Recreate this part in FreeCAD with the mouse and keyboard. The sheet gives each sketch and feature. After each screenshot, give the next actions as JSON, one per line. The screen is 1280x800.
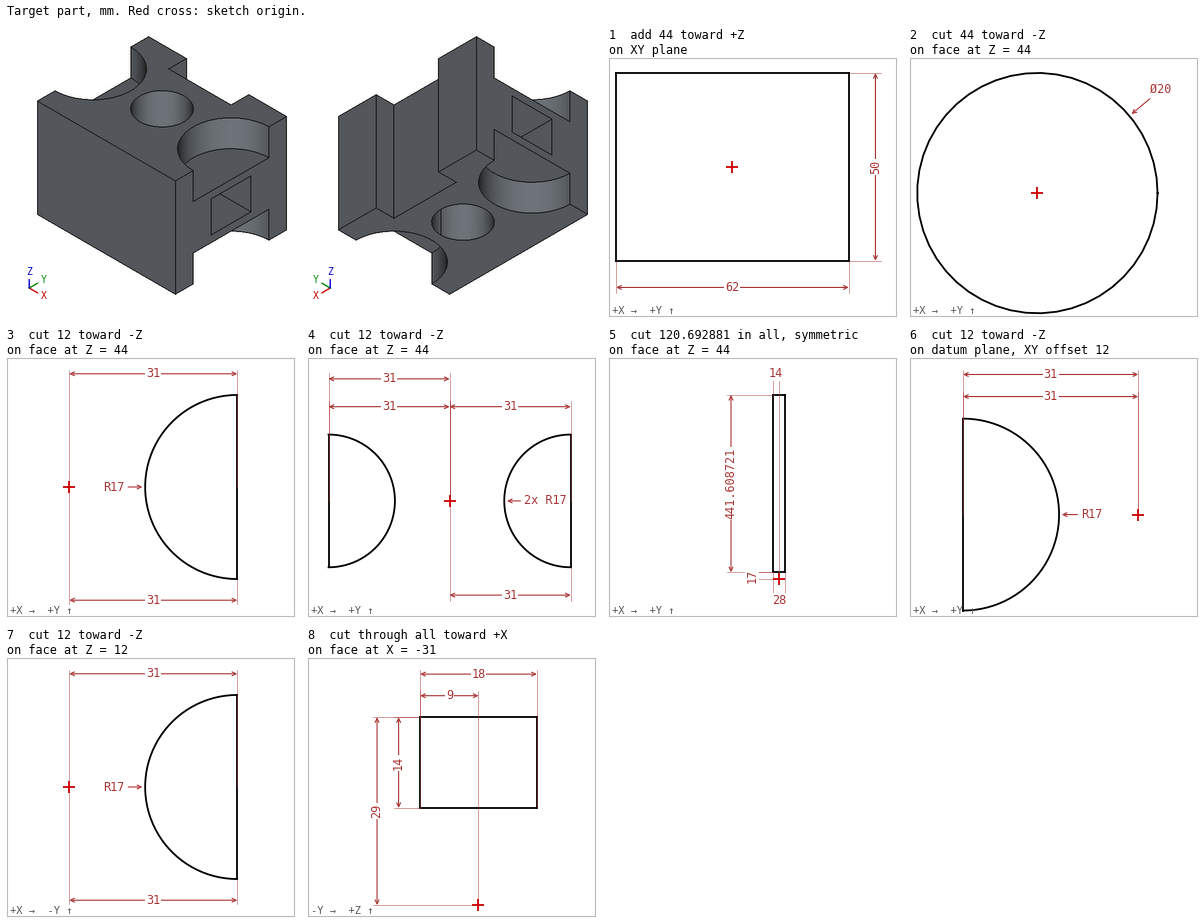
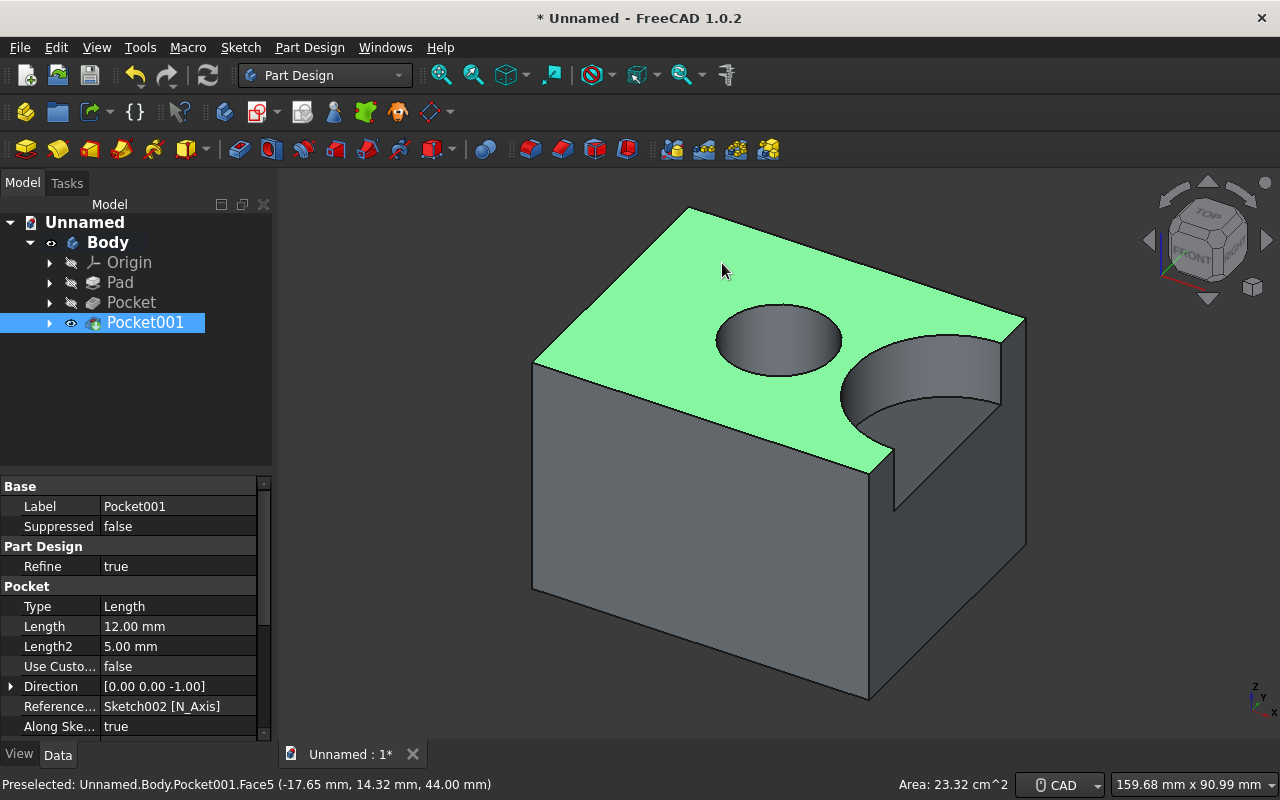
{"action": "left_click", "coordinate": [258, 112]}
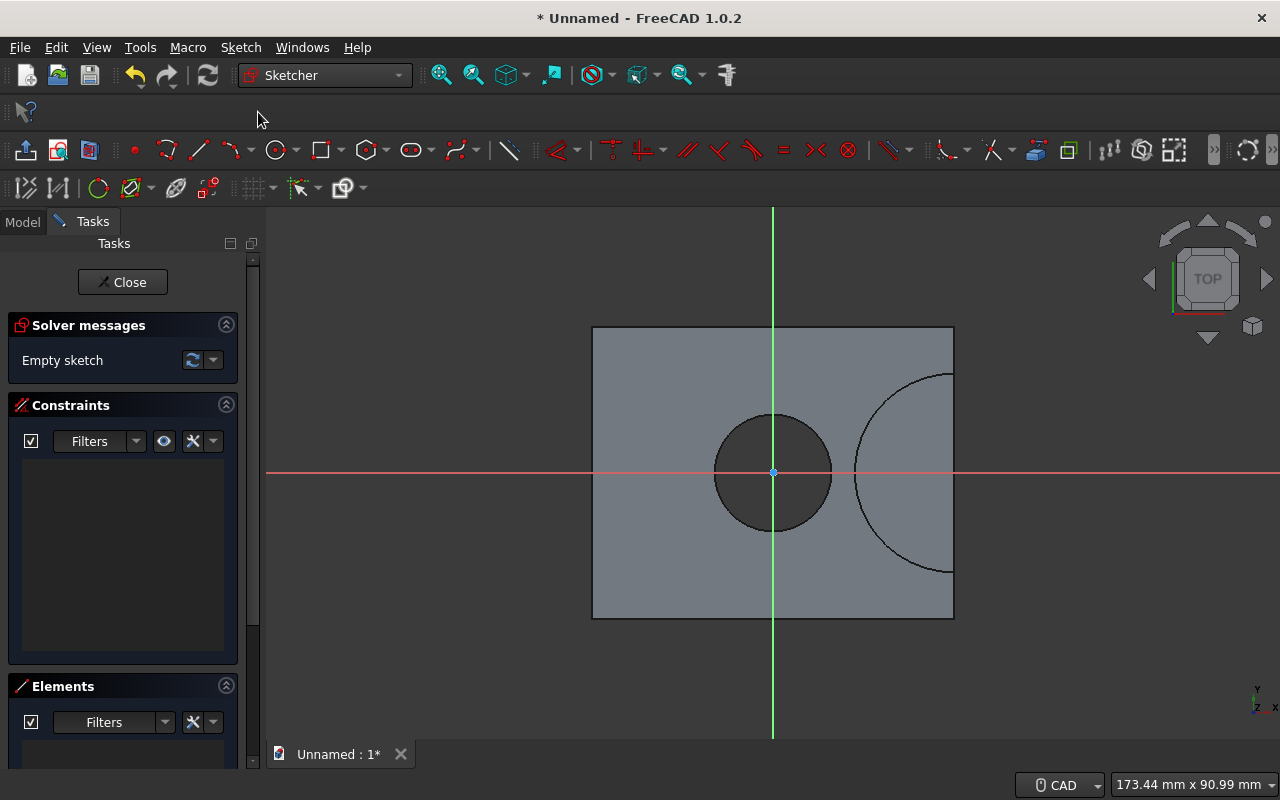
{"action": "scroll", "coordinate": [912, 473], "scroll_direction": "up", "scroll_amount": 2}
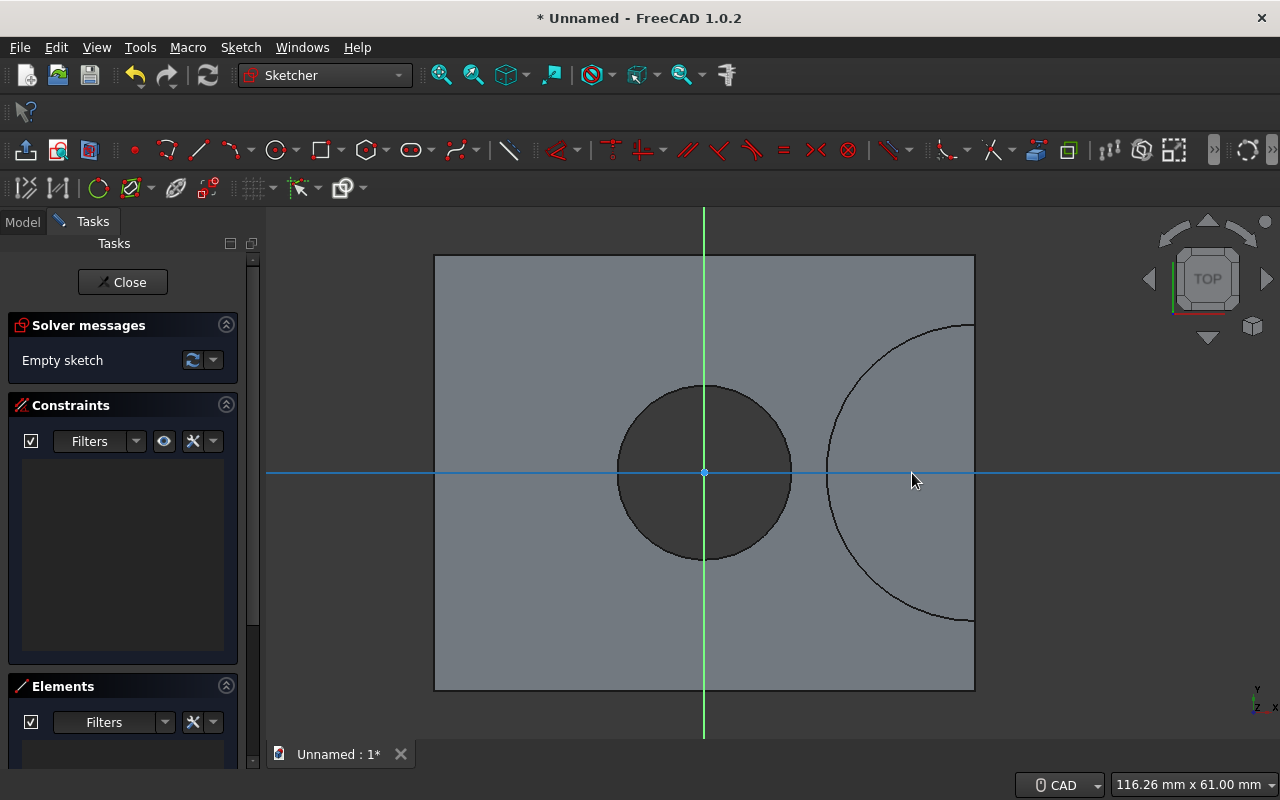
{"action": "key", "text": "g l"}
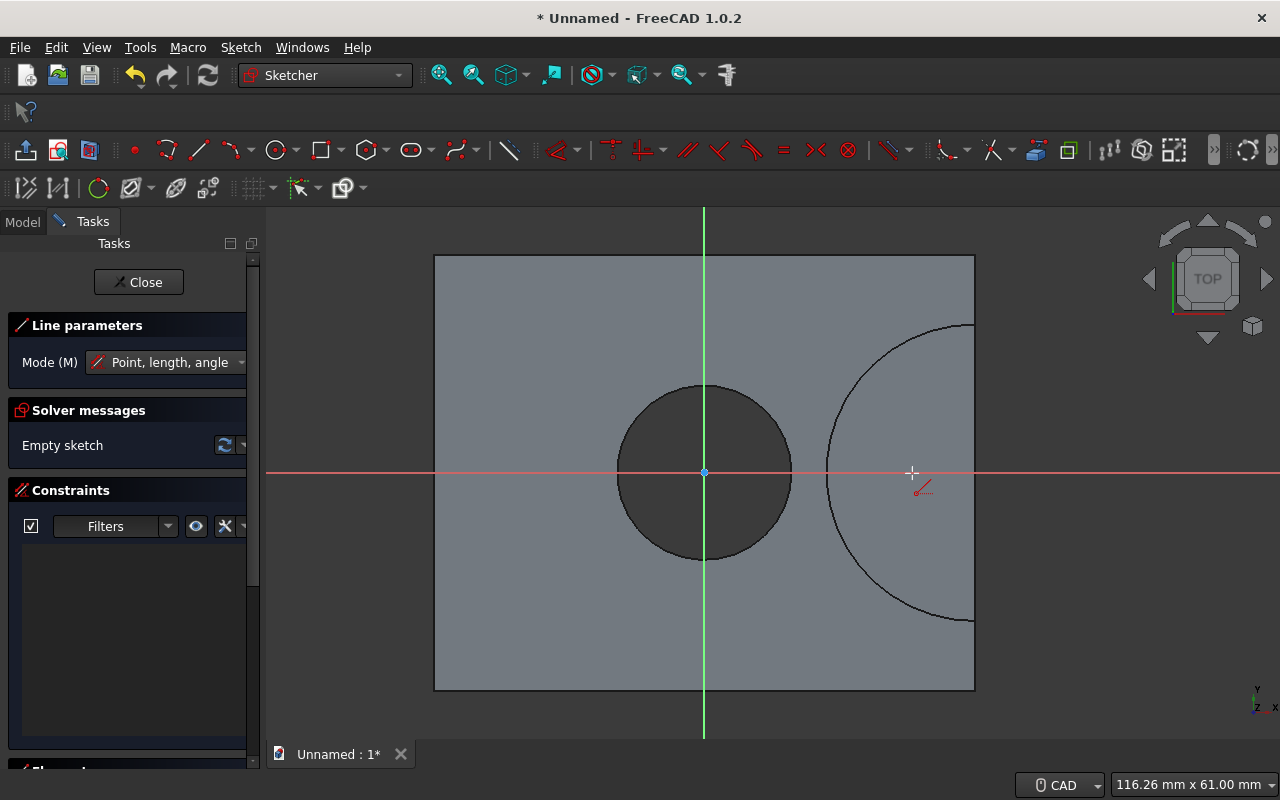
{"action": "left_click", "coordinate": [975, 621]}
{"action": "left_click", "coordinate": [975, 324]}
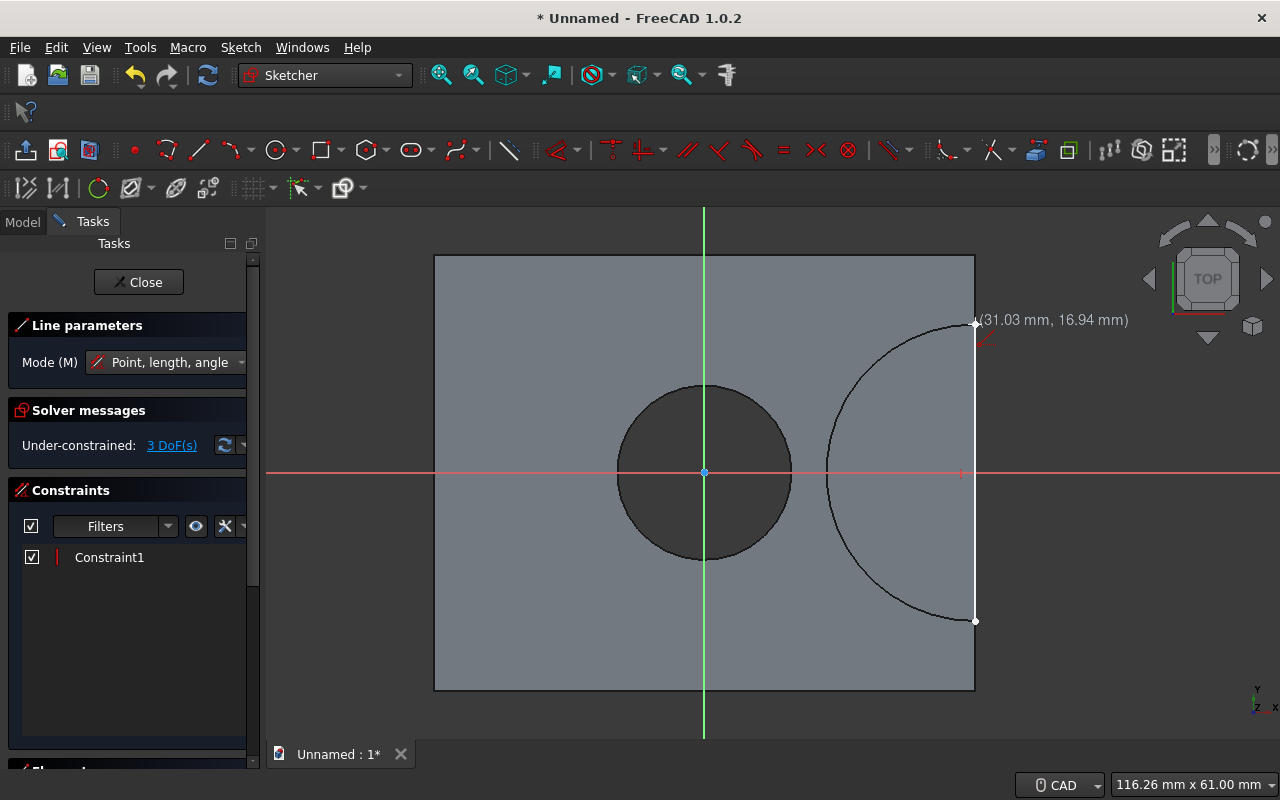
{"action": "key", "text": "g 3 a"}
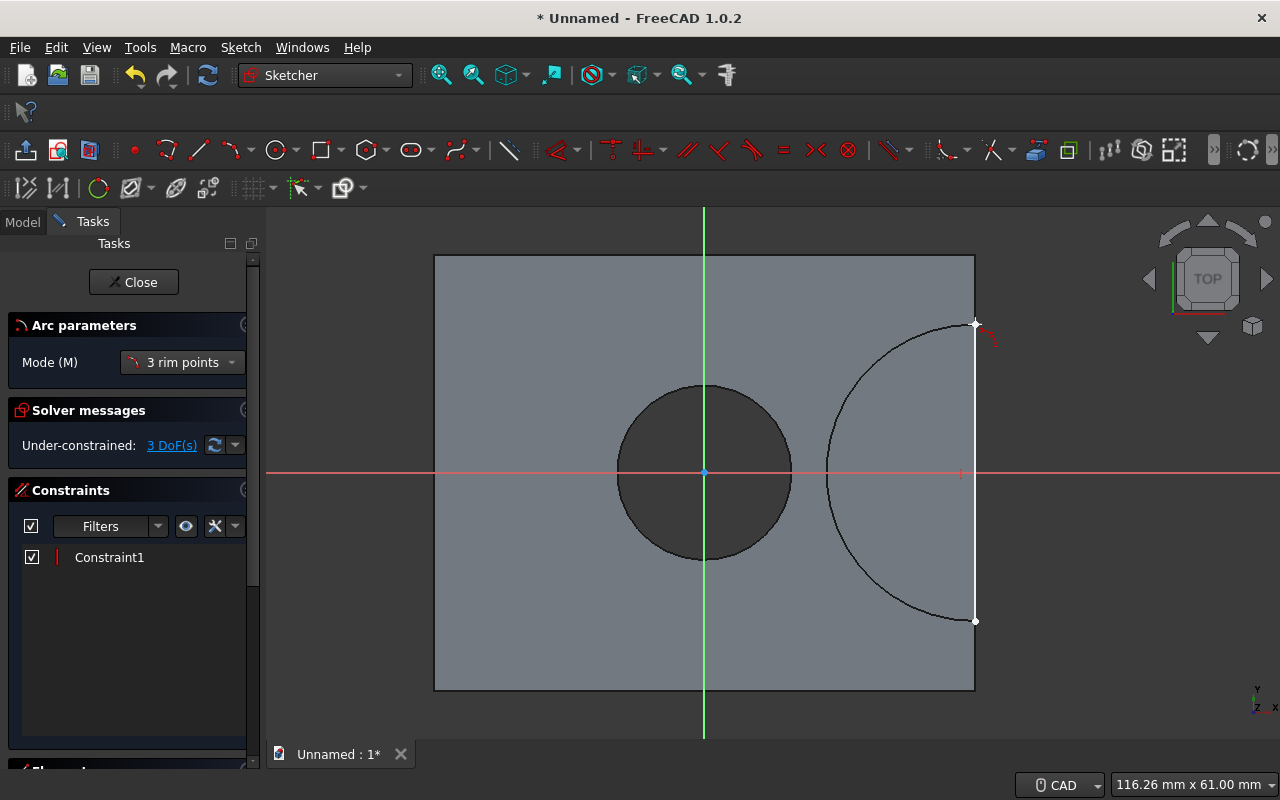
{"action": "left_click", "coordinate": [975, 325]}
{"action": "left_click", "coordinate": [975, 622]}
{"action": "left_click", "coordinate": [834, 427]}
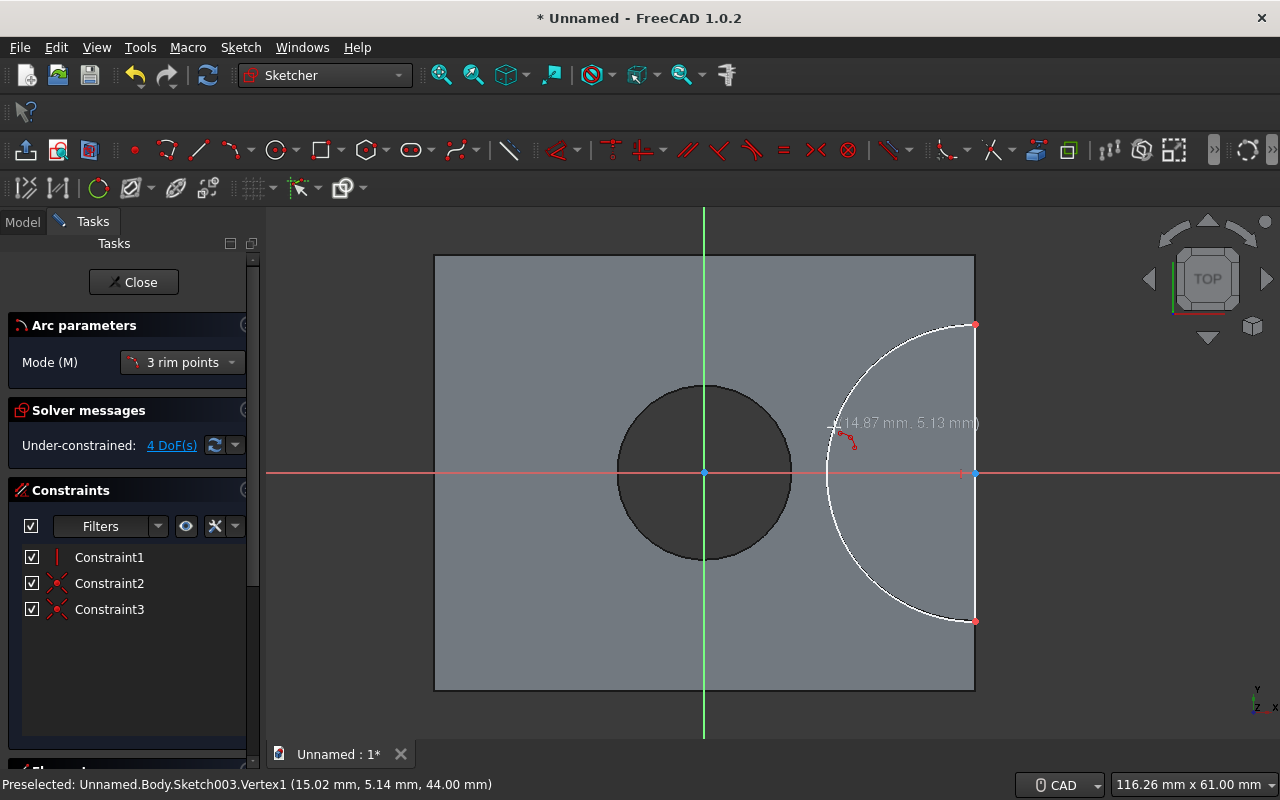
{"action": "left_click", "coordinate": [200, 150]}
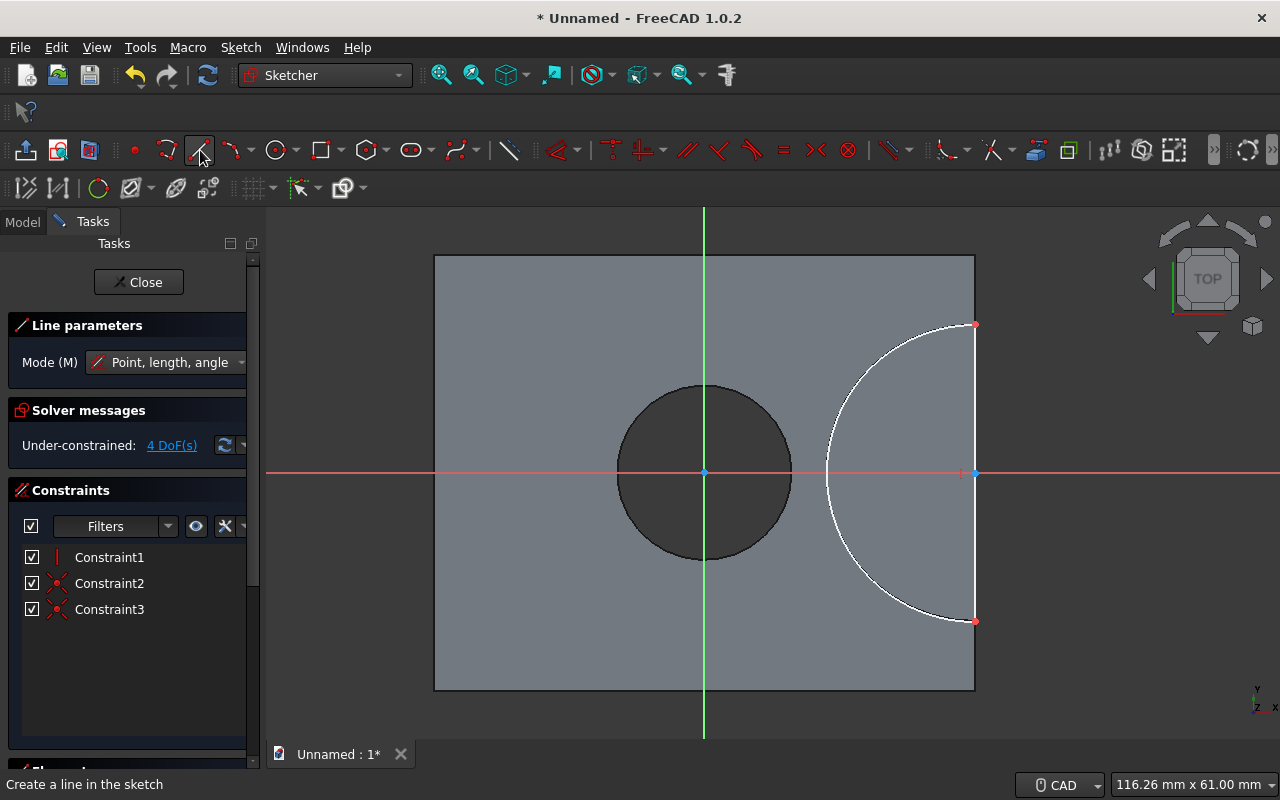
{"action": "left_click", "coordinate": [434, 324]}
{"action": "left_click", "coordinate": [434, 621]}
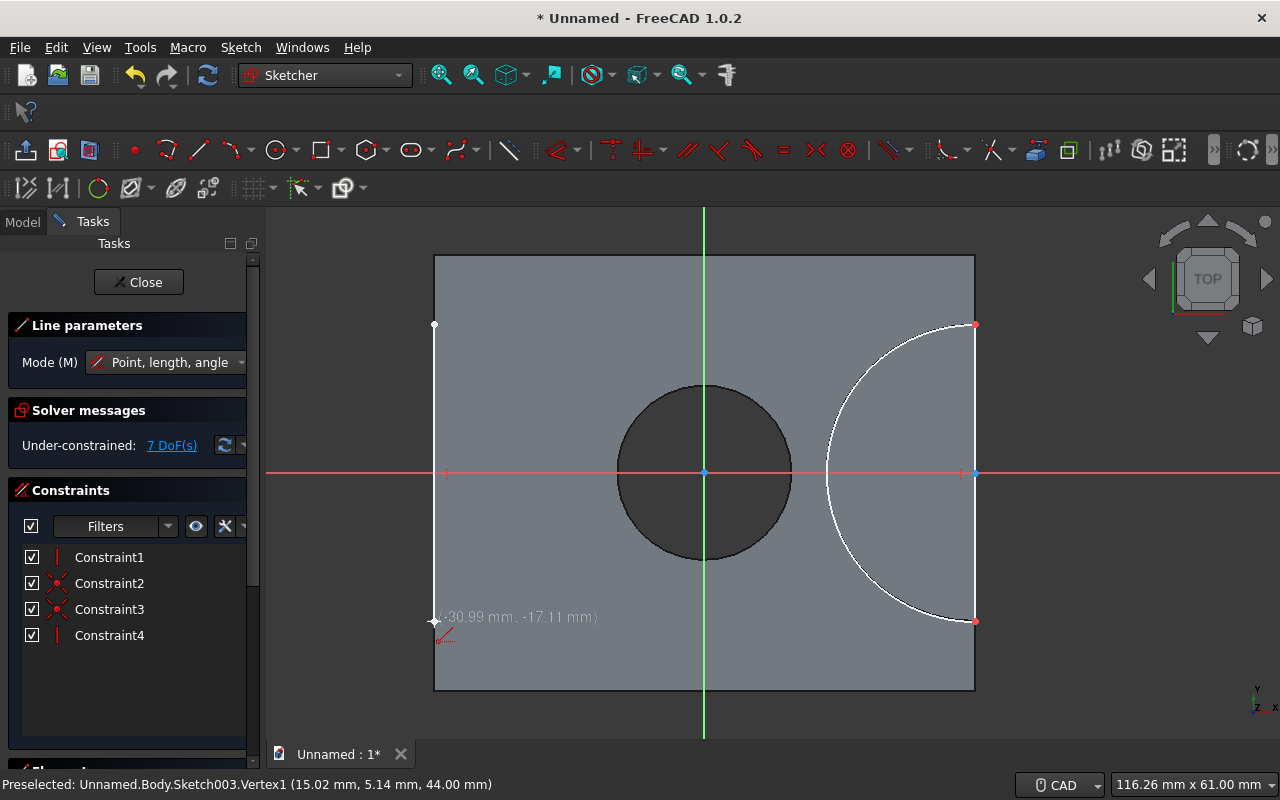
{"action": "left_click", "coordinate": [232, 150]}